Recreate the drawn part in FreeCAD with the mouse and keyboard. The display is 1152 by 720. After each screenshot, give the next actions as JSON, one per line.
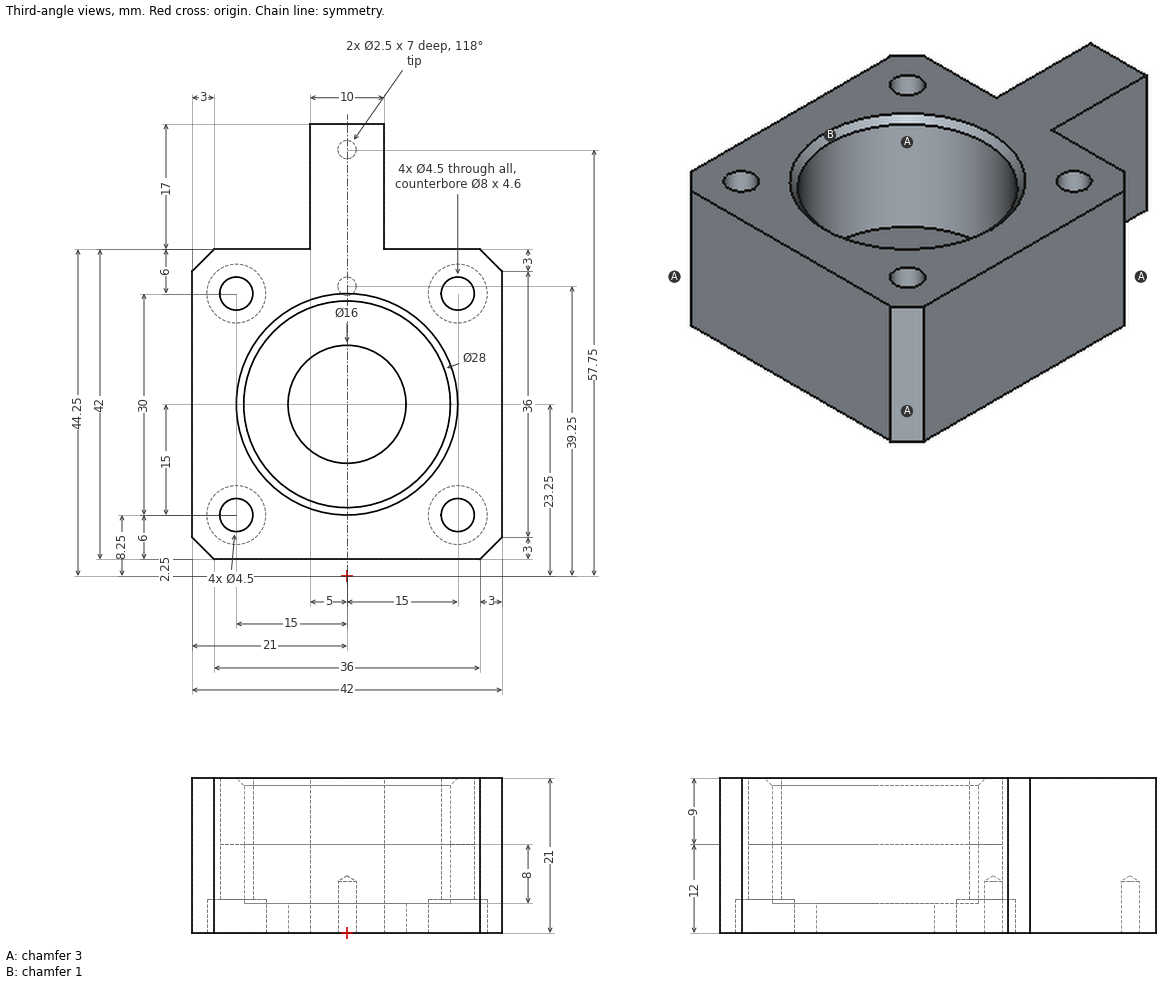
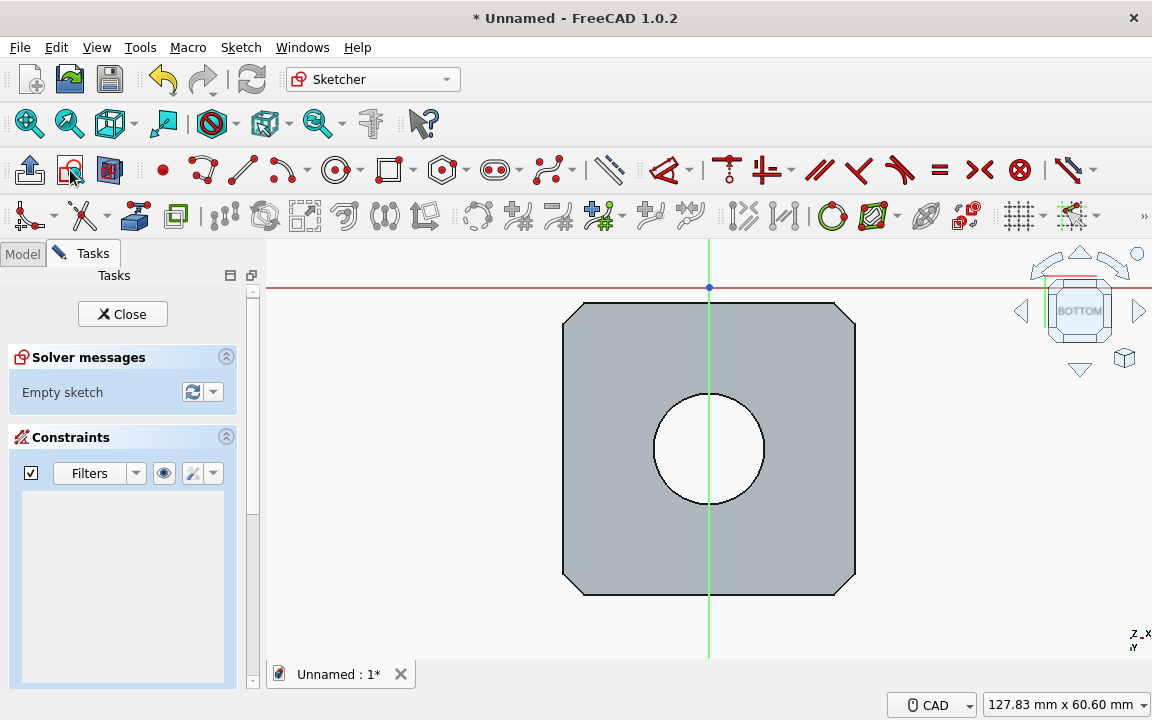
{"action": "scroll", "coordinate": [331, 543], "scroll_direction": "down", "scroll_amount": 1}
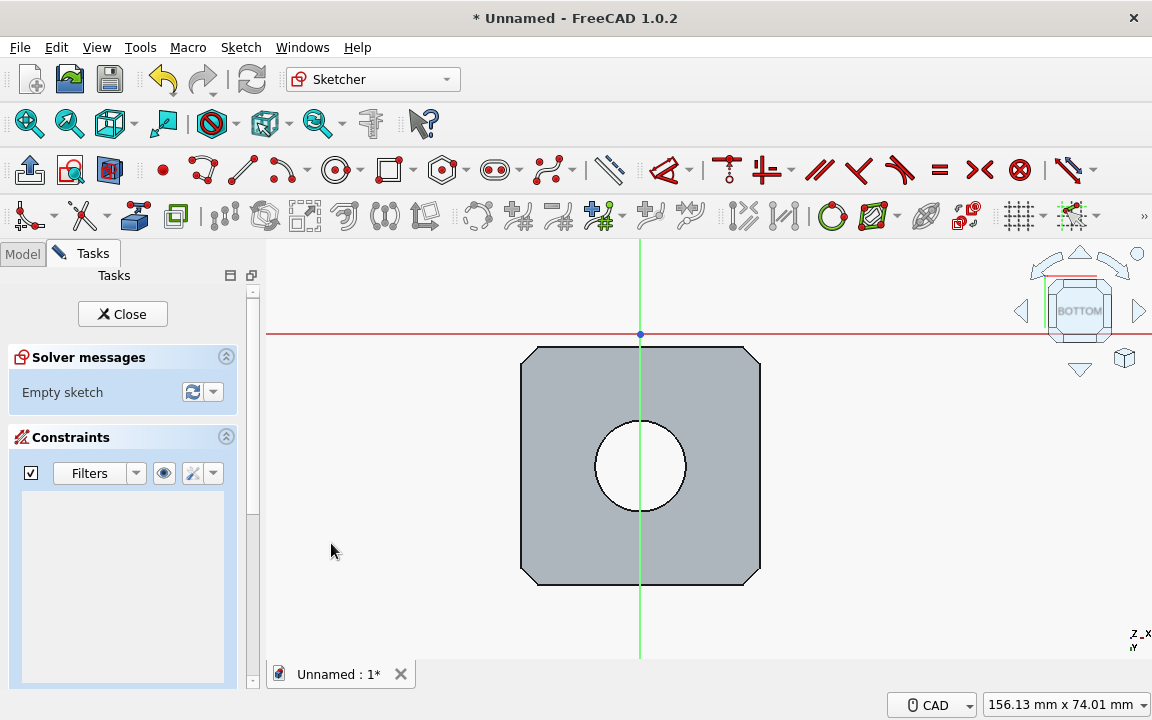
{"action": "left_click", "coordinate": [336, 170]}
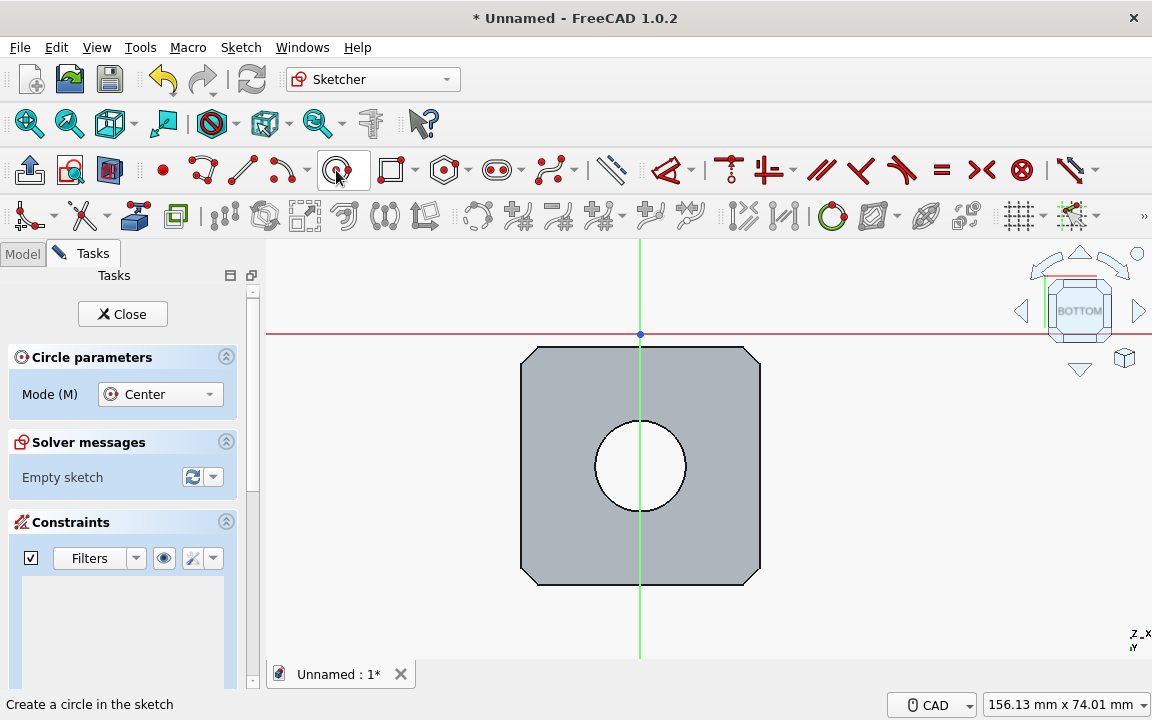
{"action": "scroll", "coordinate": [726, 551], "scroll_direction": "up", "scroll_amount": 3}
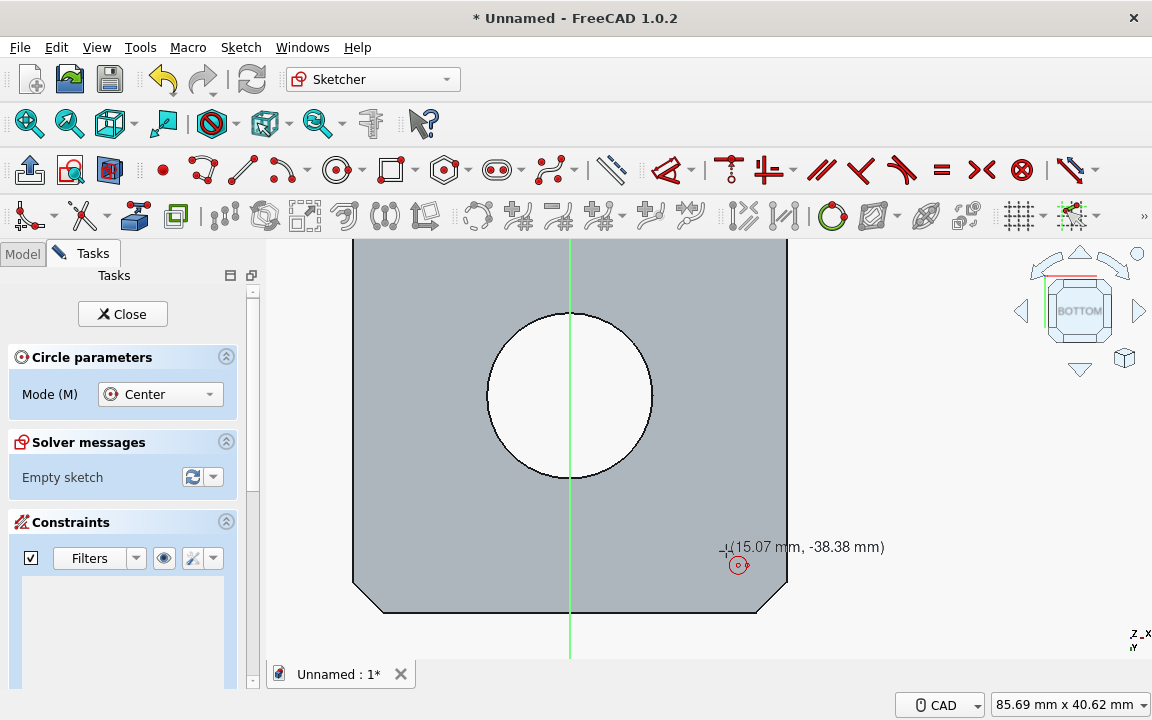
{"action": "left_click", "coordinate": [725, 551]}
{"action": "left_click", "coordinate": [741, 534]}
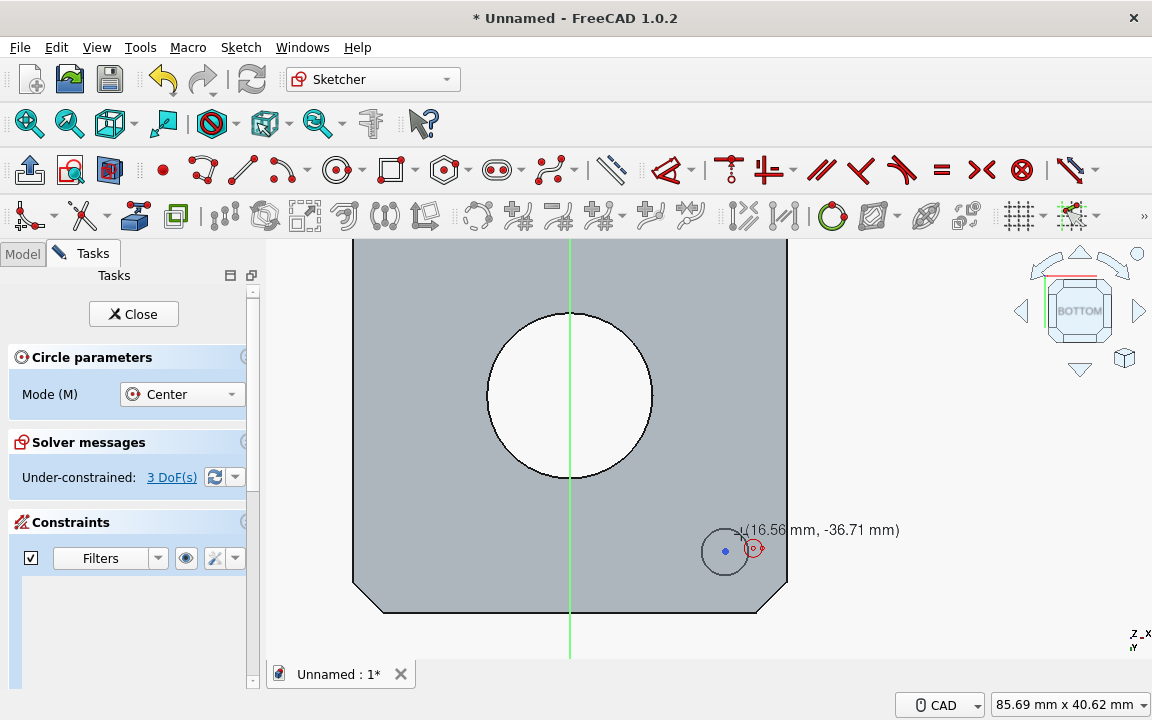
{"action": "left_click", "coordinate": [415, 551]}
{"action": "left_click", "coordinate": [431, 534]}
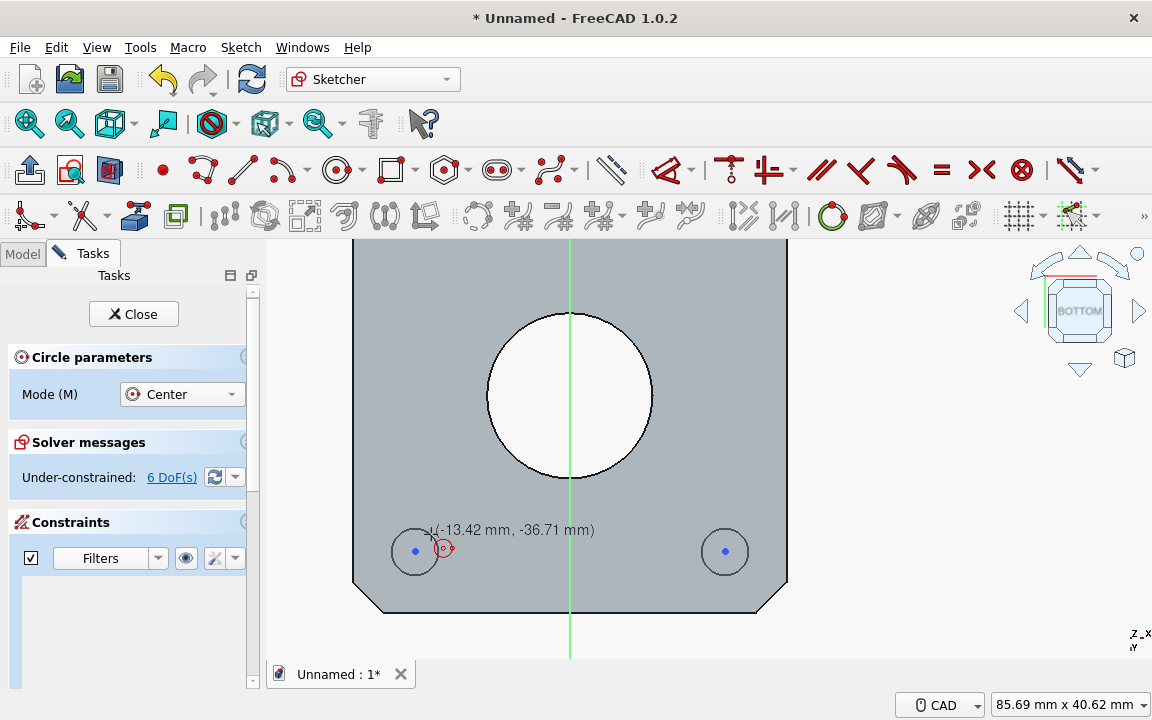
{"action": "scroll", "coordinate": [784, 620], "scroll_direction": "down", "scroll_amount": 2}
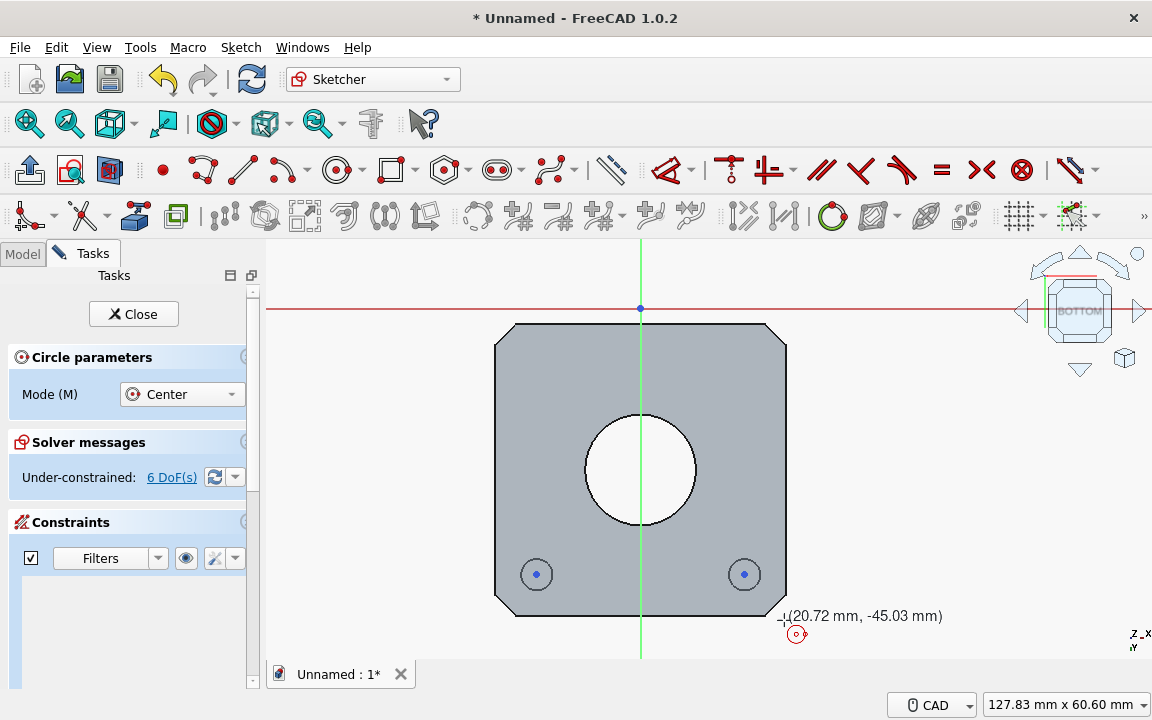
{"action": "scroll", "coordinate": [537, 366], "scroll_direction": "up", "scroll_amount": 2}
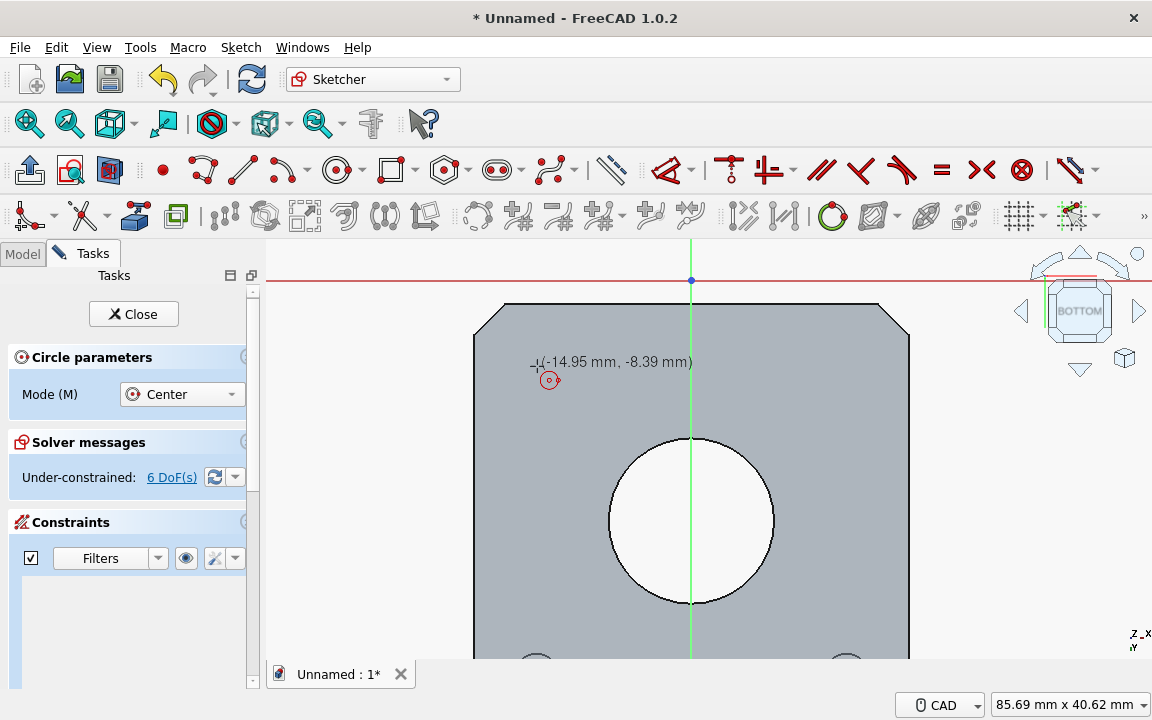
{"action": "left_click", "coordinate": [536, 366]}
{"action": "left_click", "coordinate": [553, 349]}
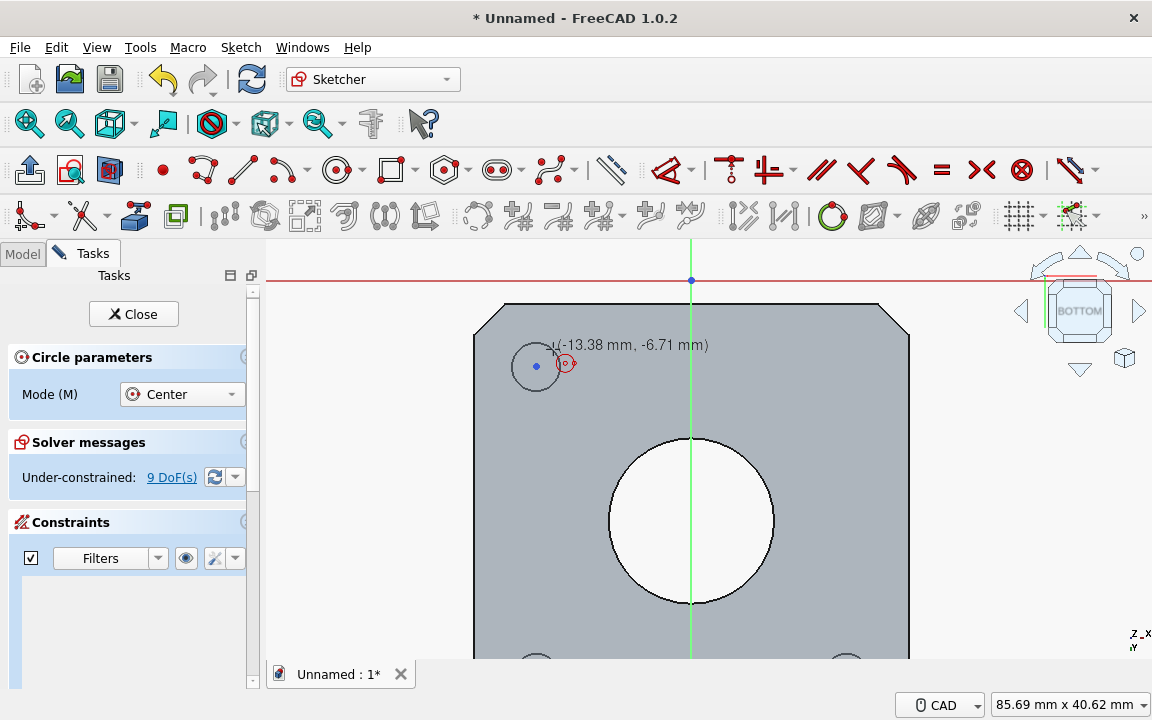
{"action": "left_click", "coordinate": [846, 366]}
{"action": "left_click", "coordinate": [863, 349]}
{"action": "key", "text": "Escape"}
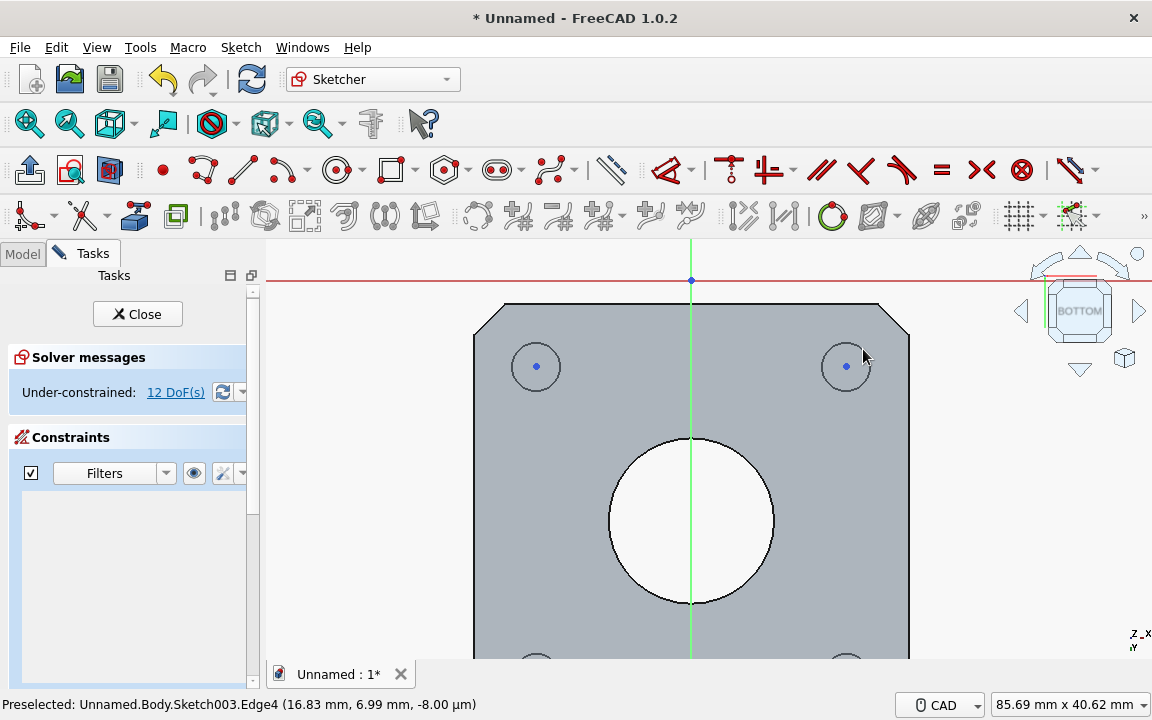
{"action": "scroll", "coordinate": [537, 366], "scroll_direction": "down", "scroll_amount": 2}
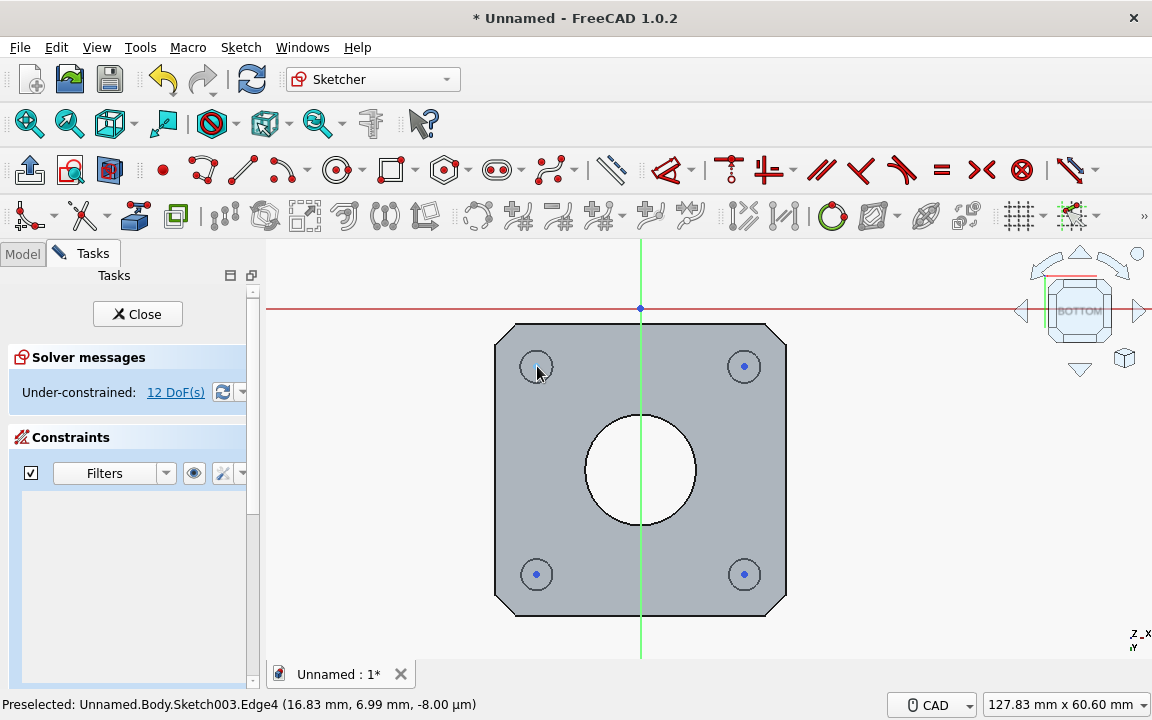
{"action": "left_click", "coordinate": [756, 564]}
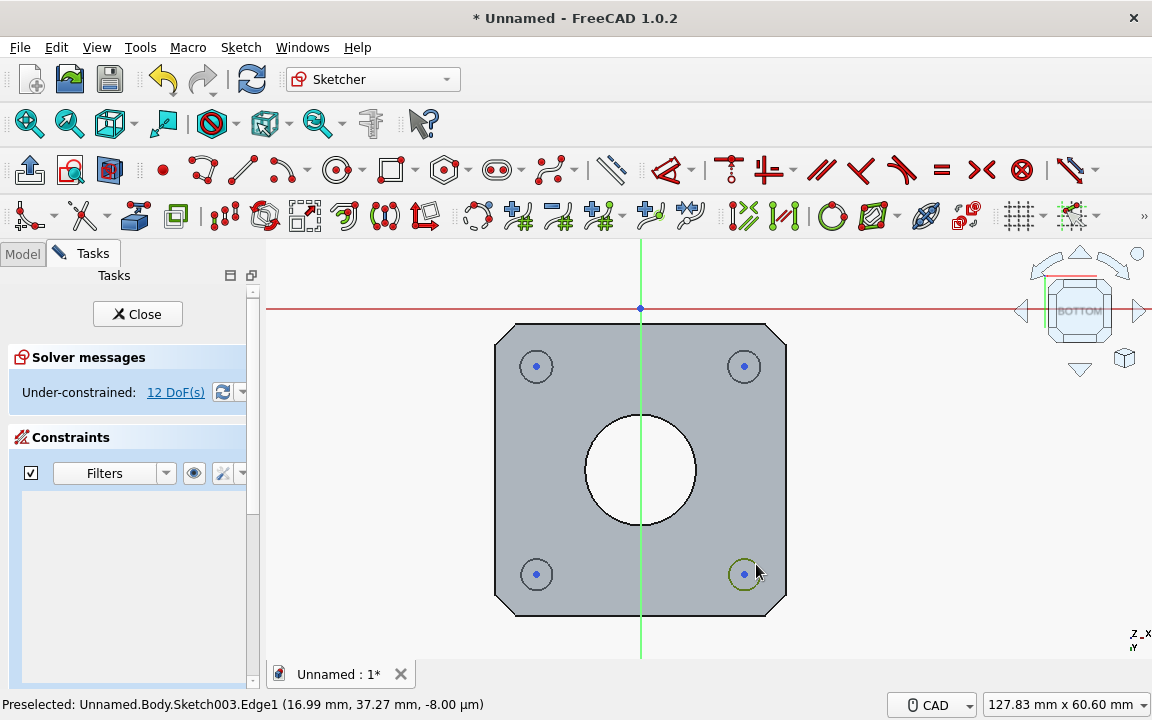
{"action": "left_click", "coordinate": [548, 564]}